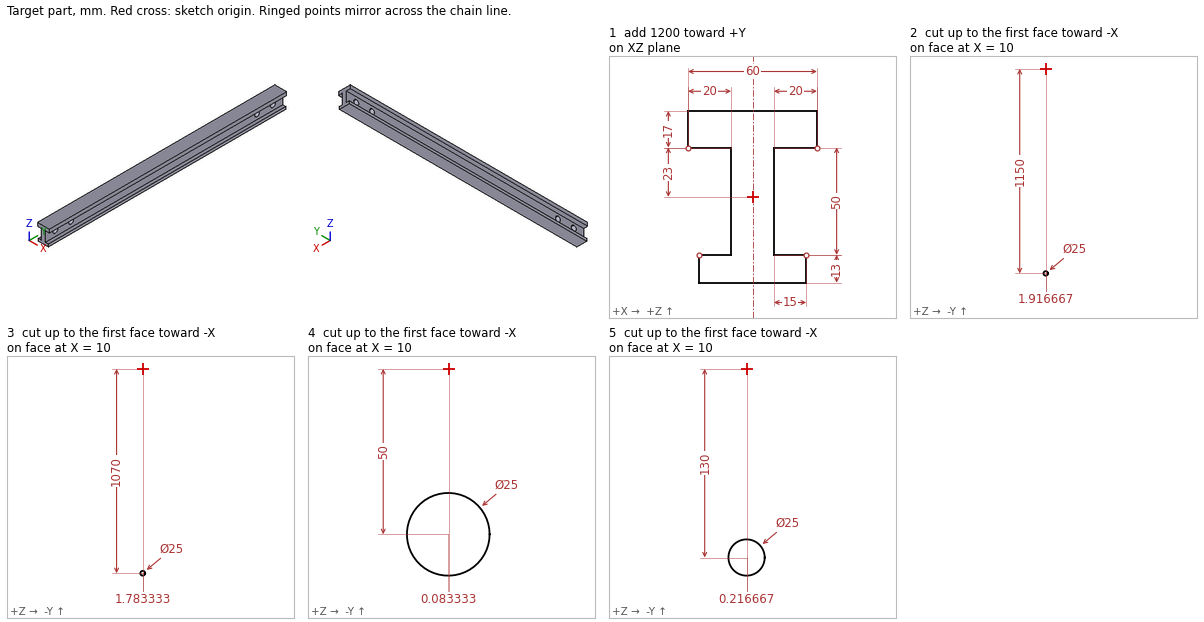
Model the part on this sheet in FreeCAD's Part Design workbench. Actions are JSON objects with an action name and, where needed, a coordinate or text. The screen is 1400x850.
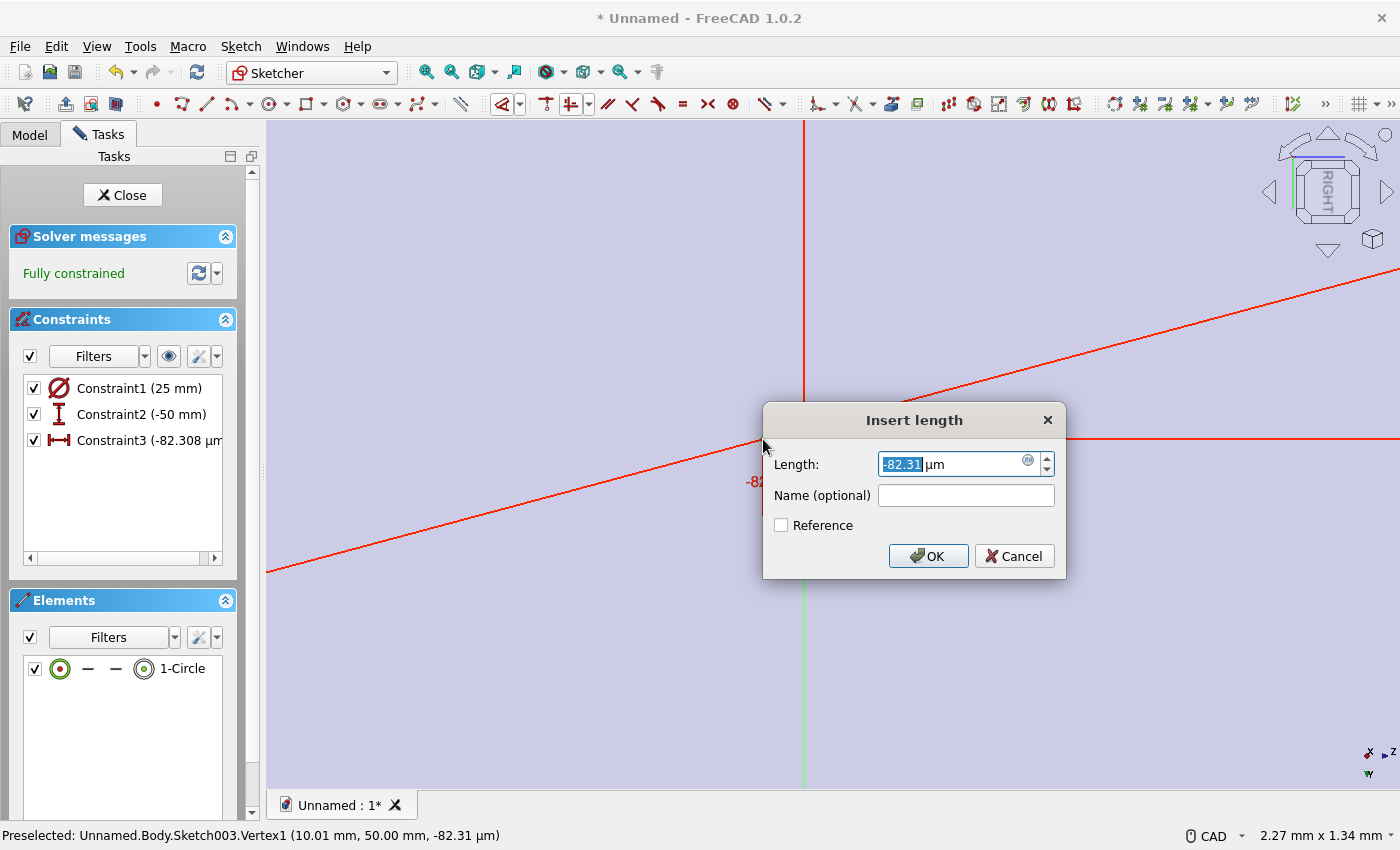
{"action": "key", "text": "ctrl+a"}
{"action": "type", "text": "-0.083333 mm"}
{"action": "key", "text": "Return"}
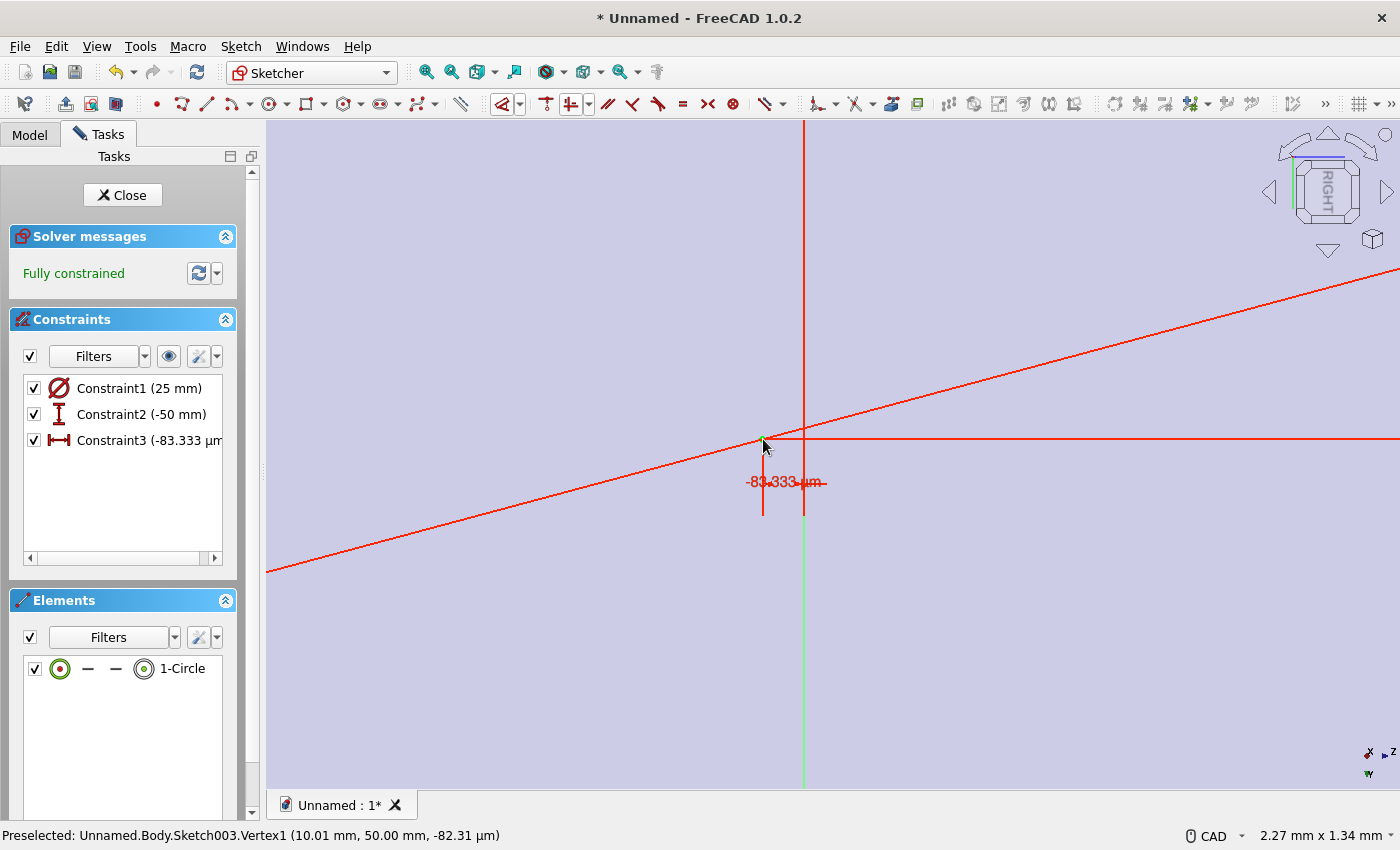
{"action": "left_click", "coordinate": [123, 195]}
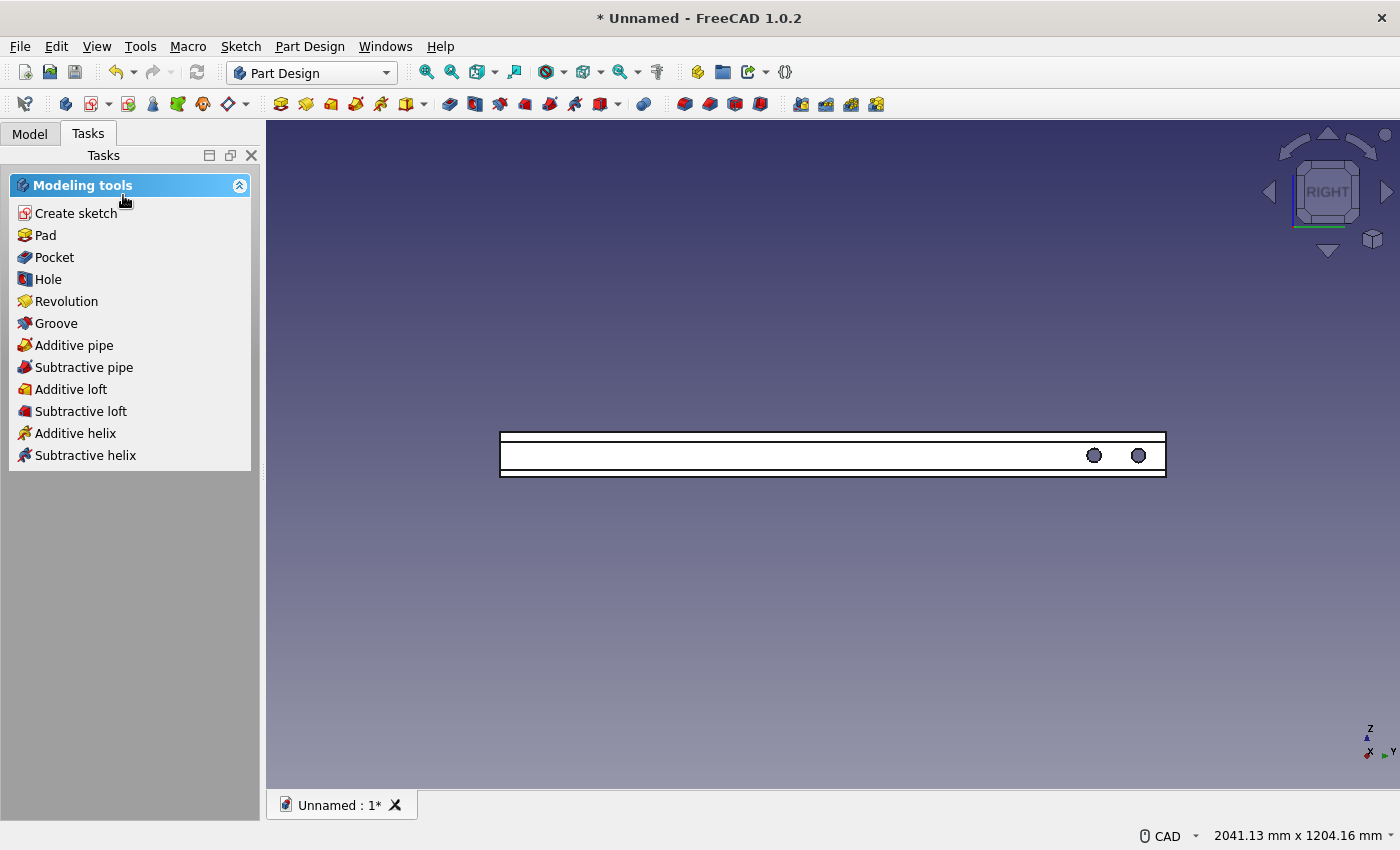
{"action": "left_click", "coordinate": [450, 104]}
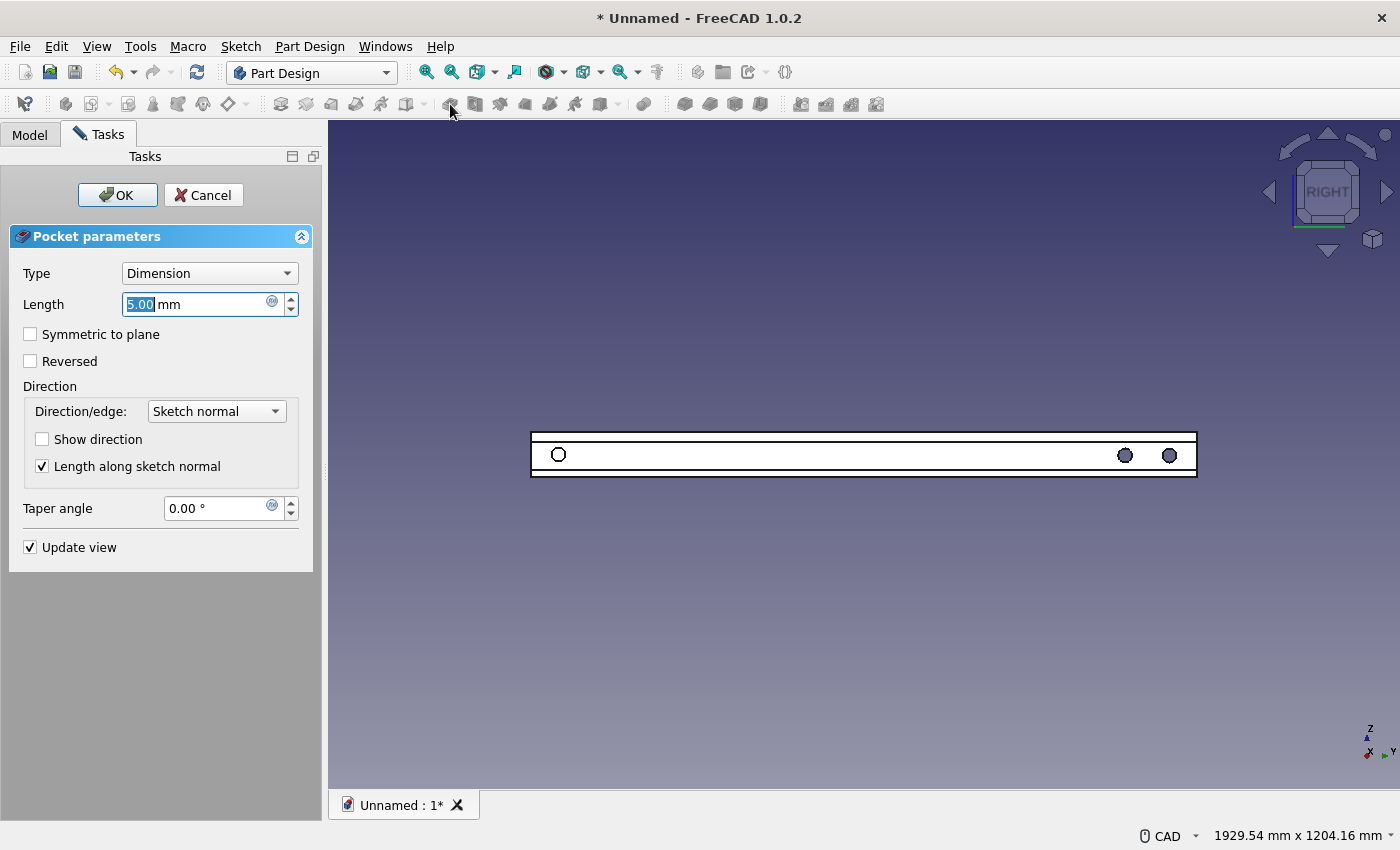
{"action": "left_click", "coordinate": [210, 274]}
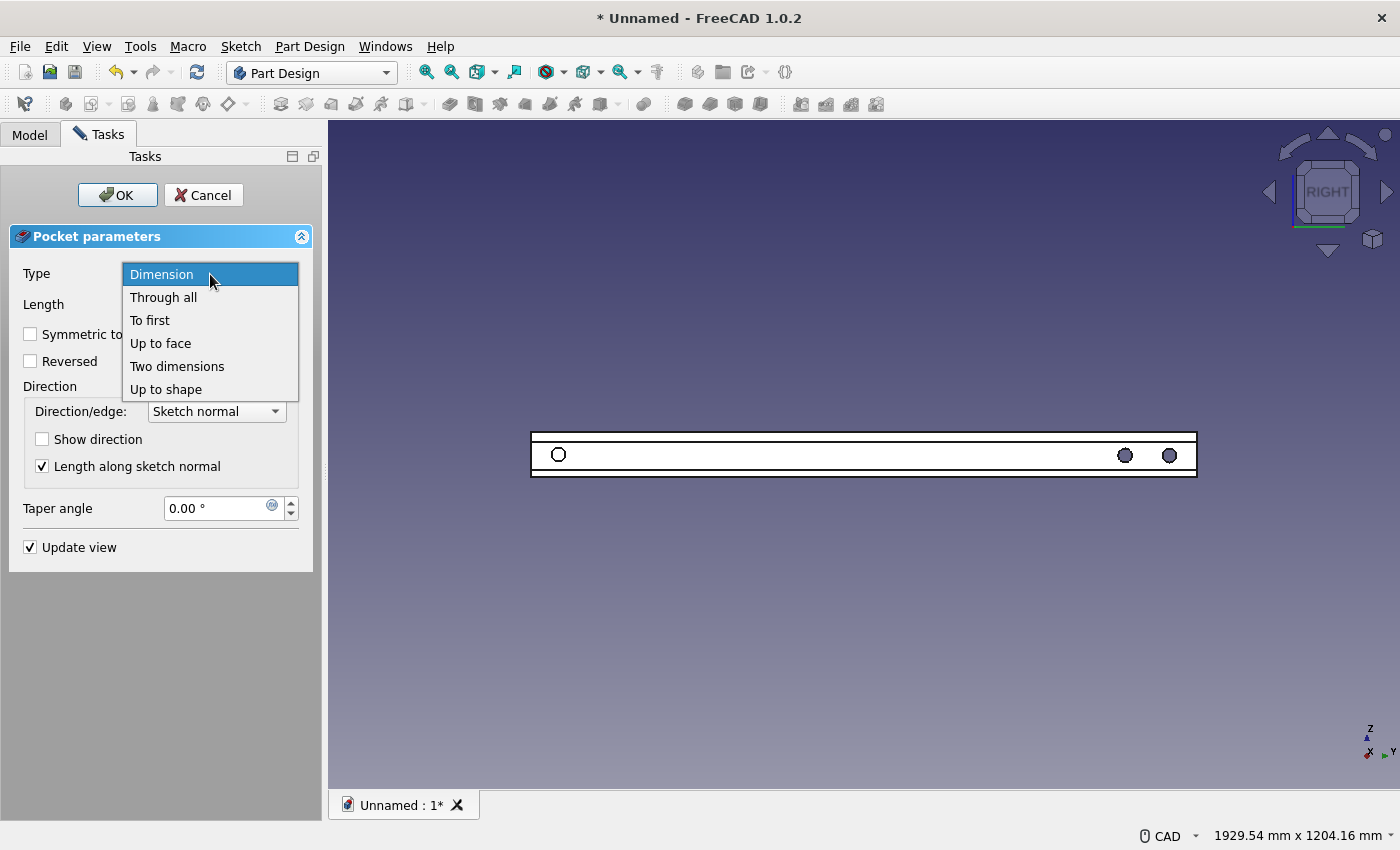
{"action": "left_click", "coordinate": [208, 320]}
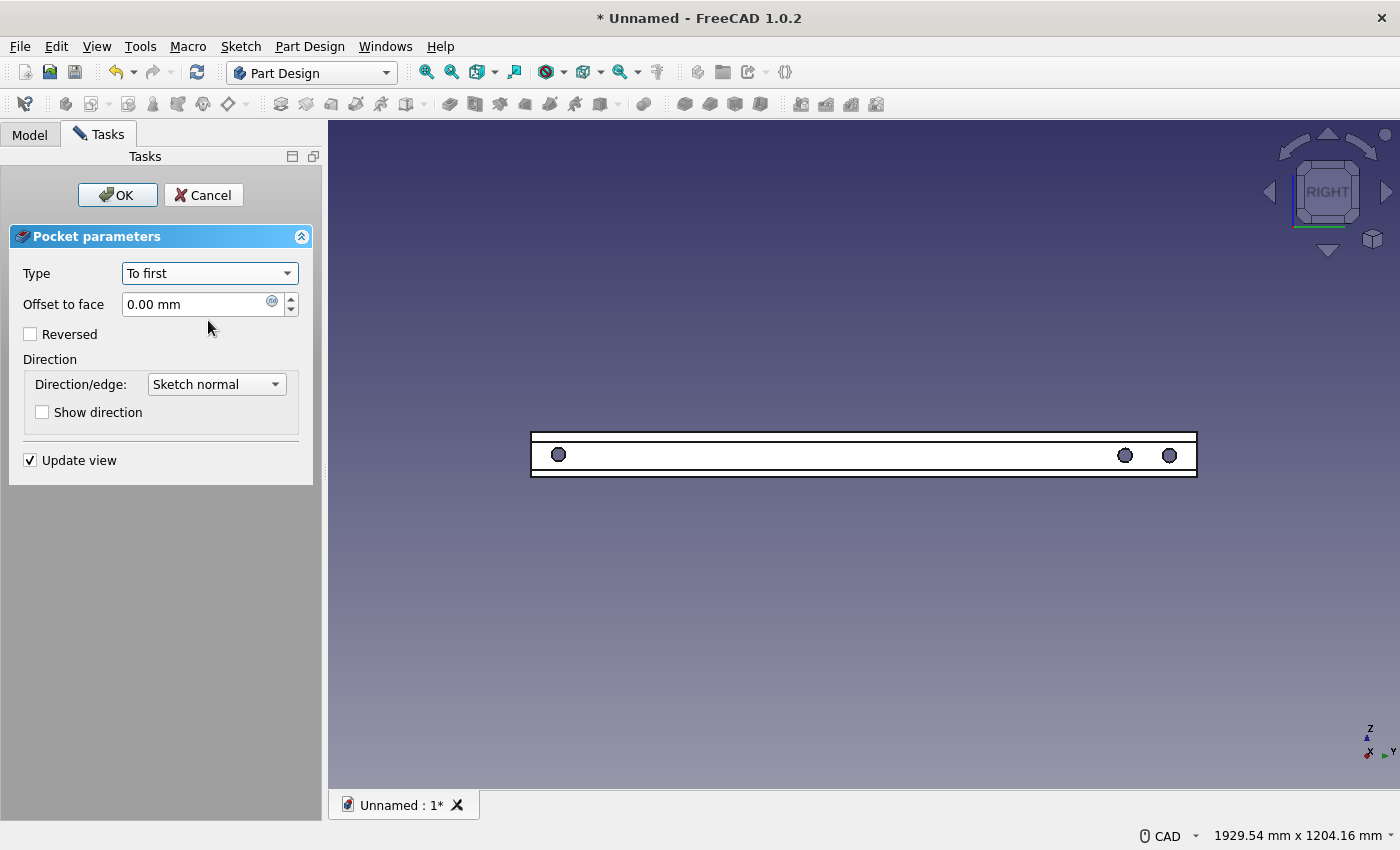
{"action": "left_click", "coordinate": [118, 195]}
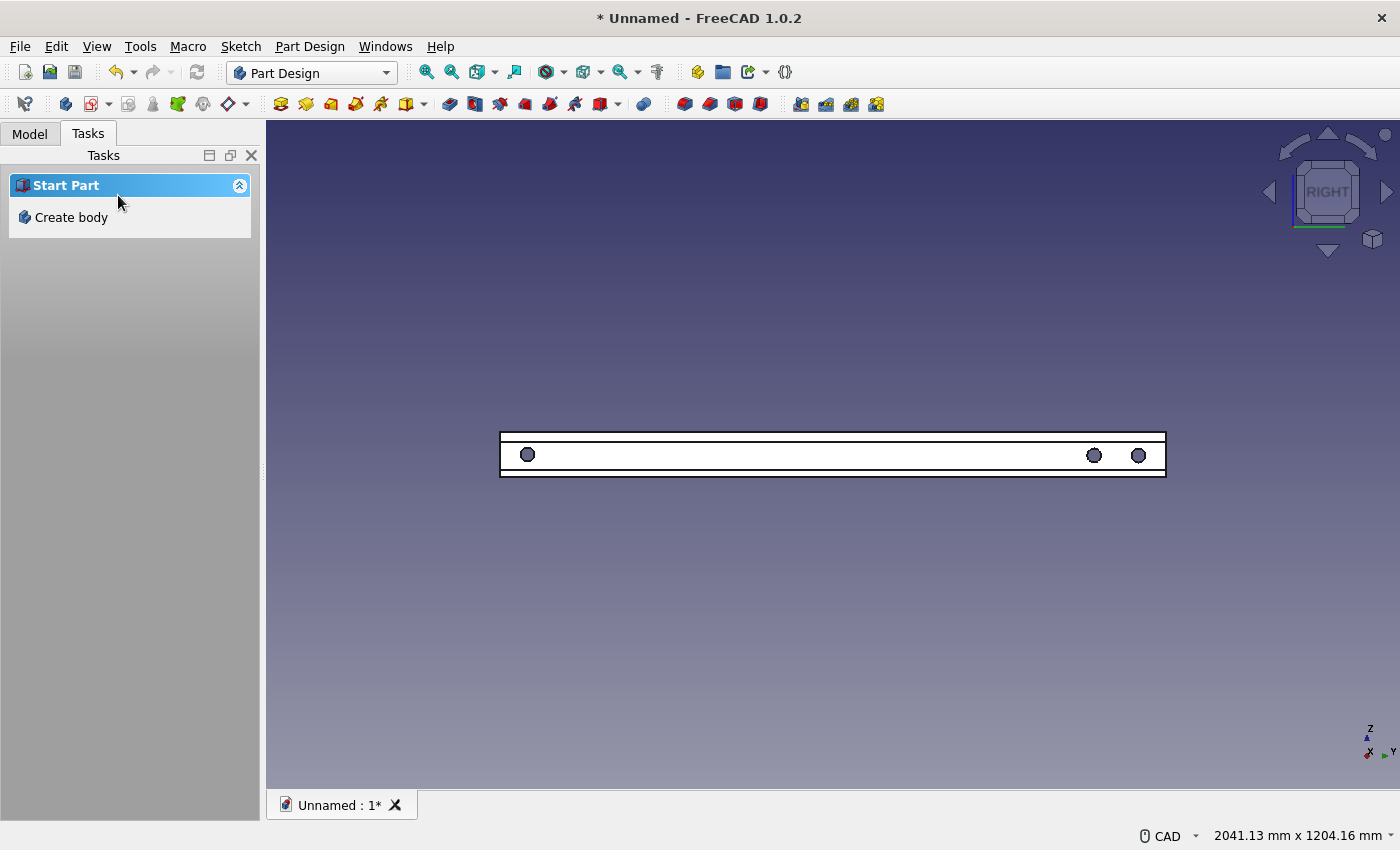
{"action": "left_click", "coordinate": [1023, 455]}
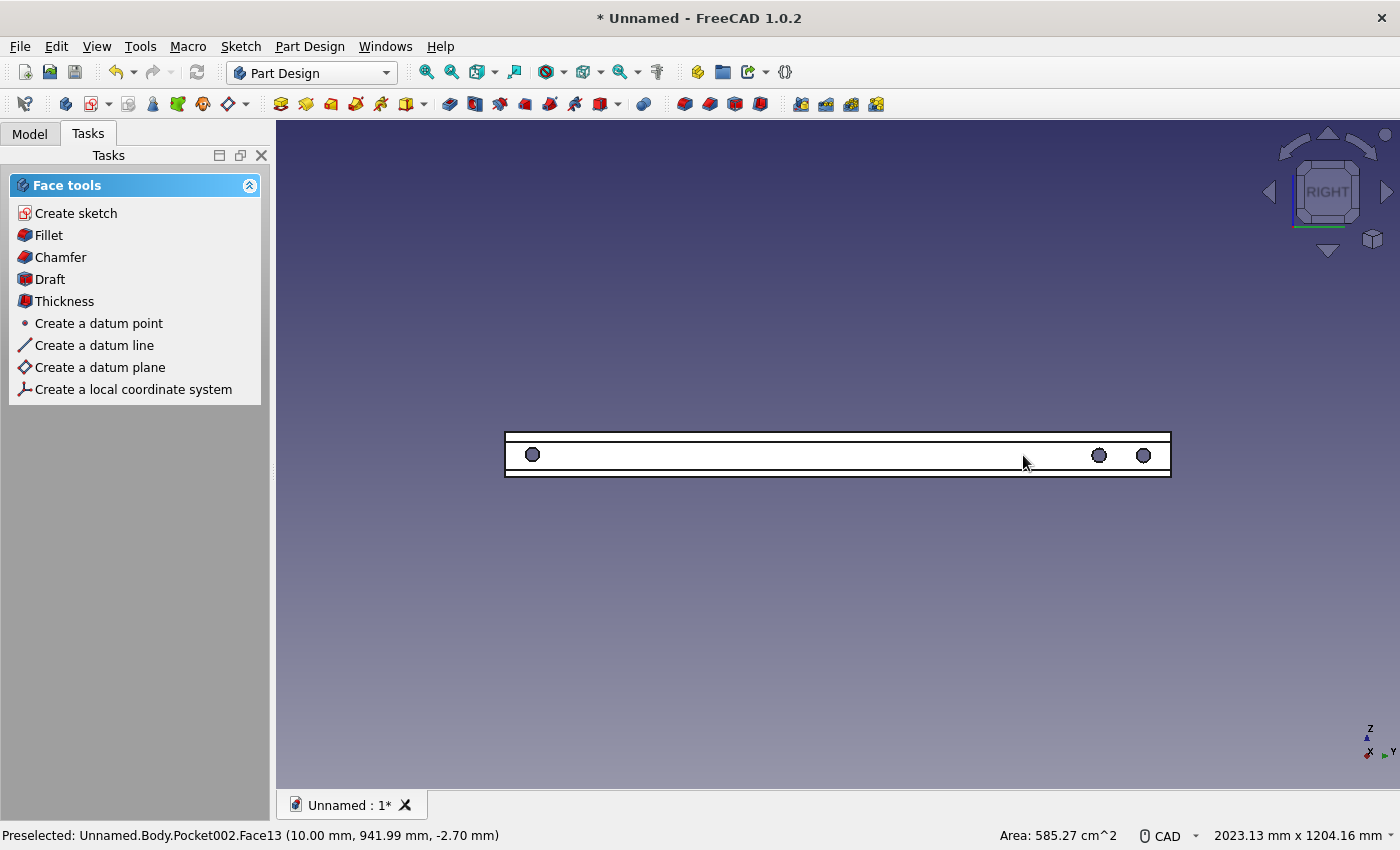
{"action": "left_click", "coordinate": [90, 104]}